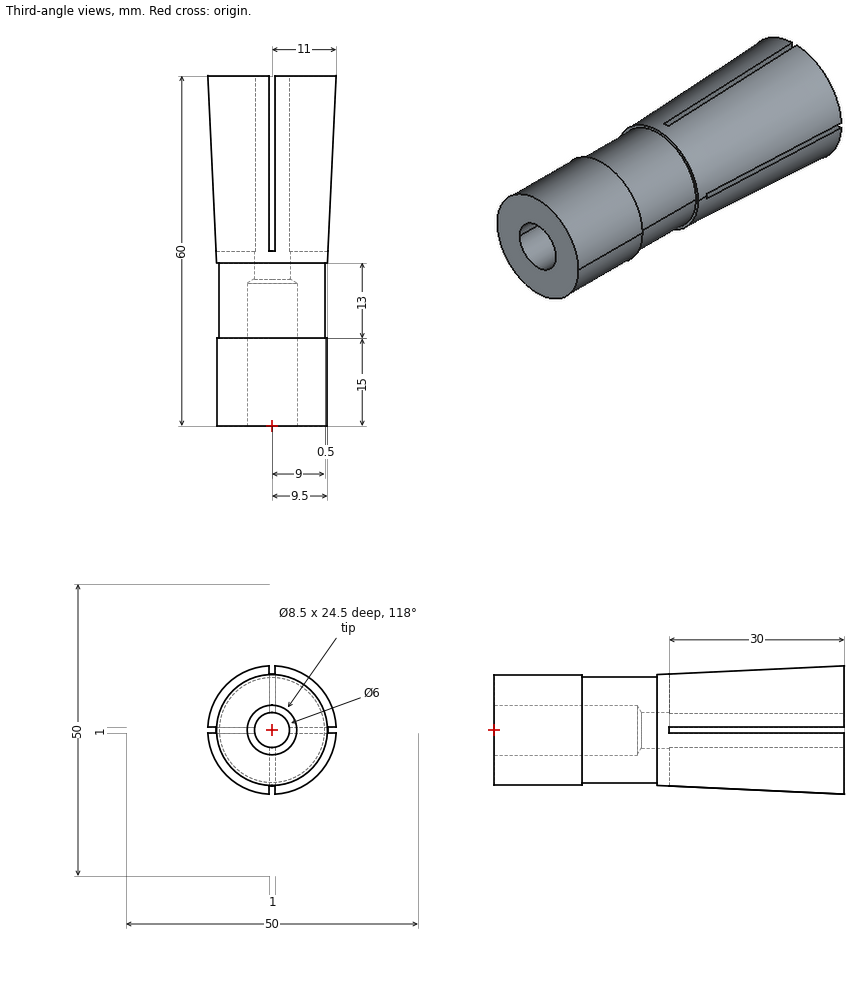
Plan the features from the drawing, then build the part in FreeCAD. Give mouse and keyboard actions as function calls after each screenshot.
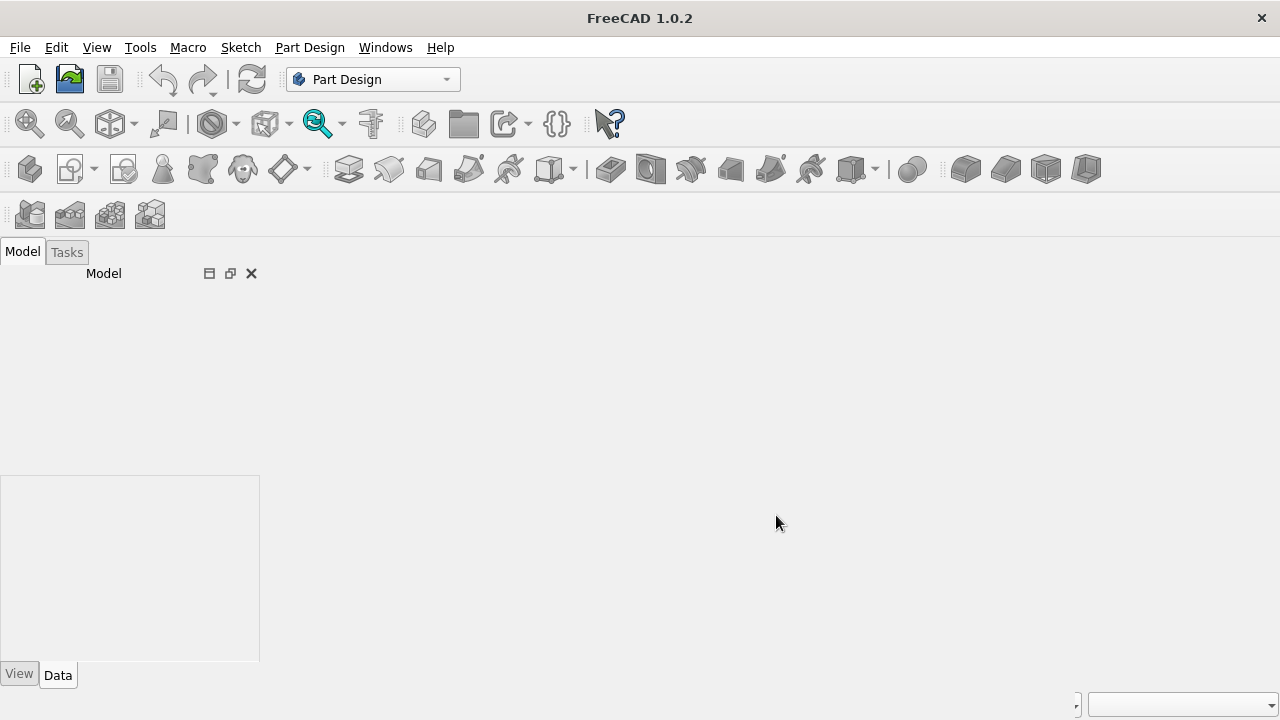
click(30, 80)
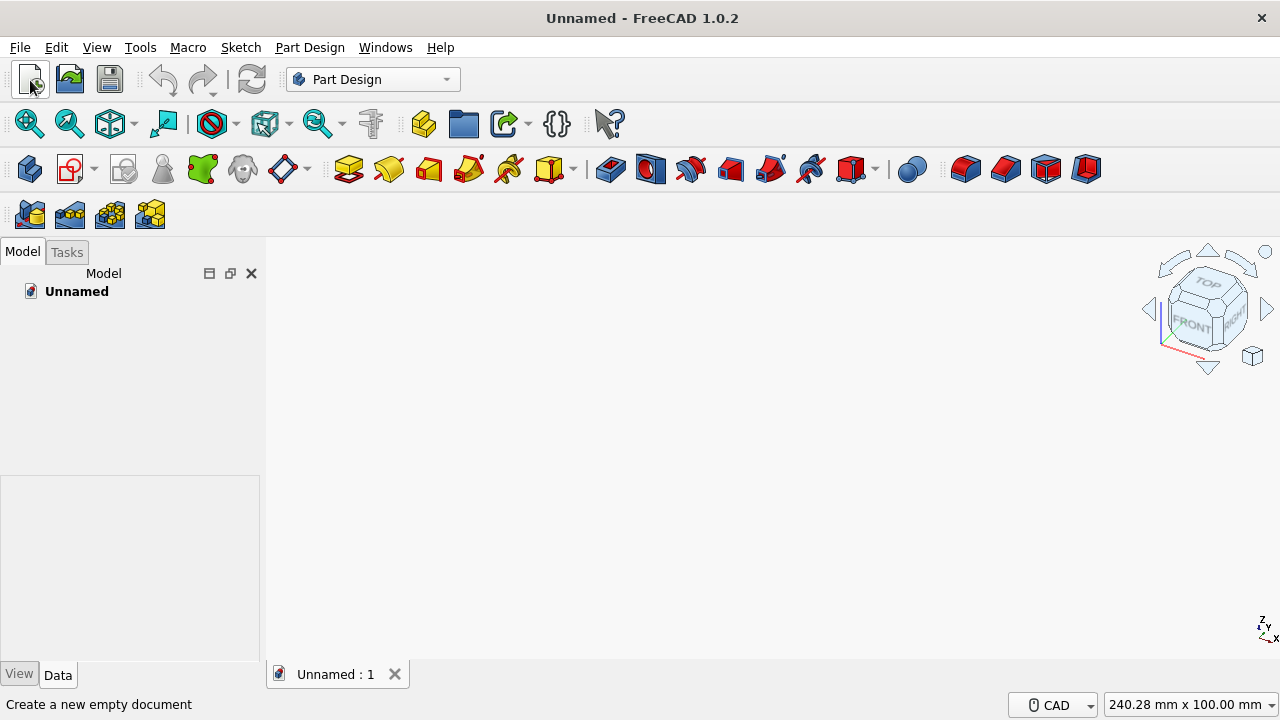
click(70, 170)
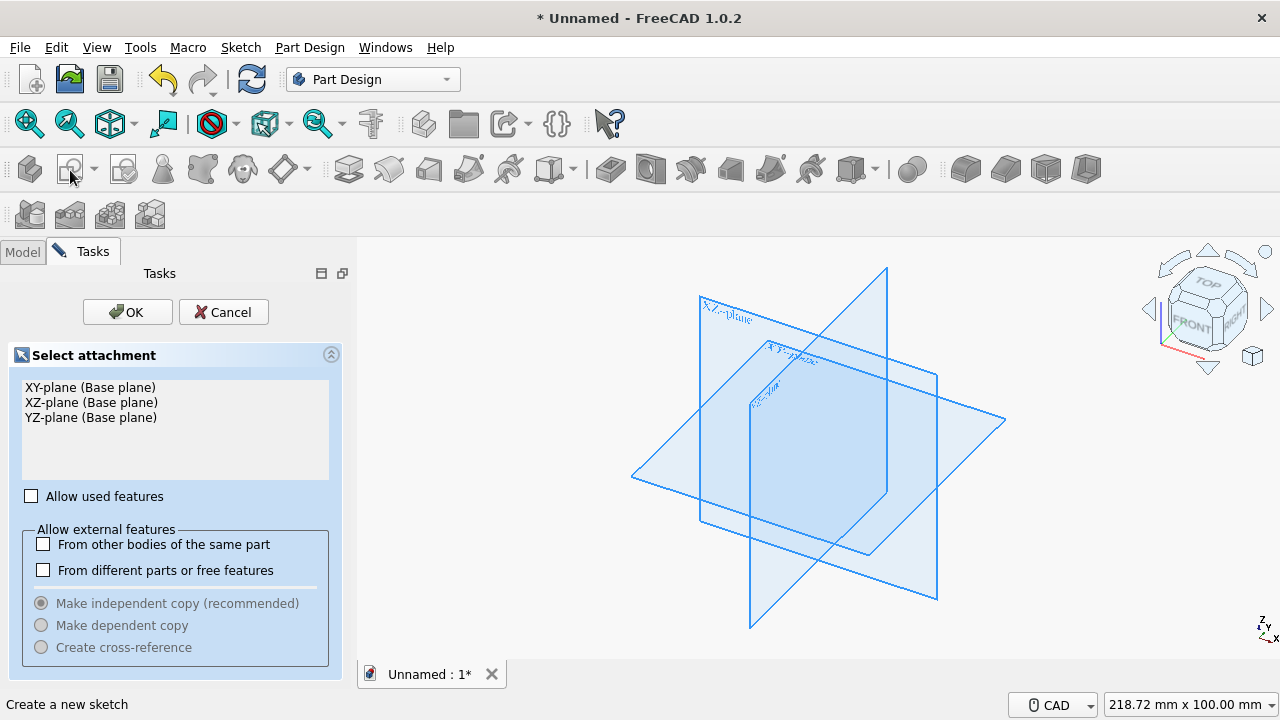
click(82, 388)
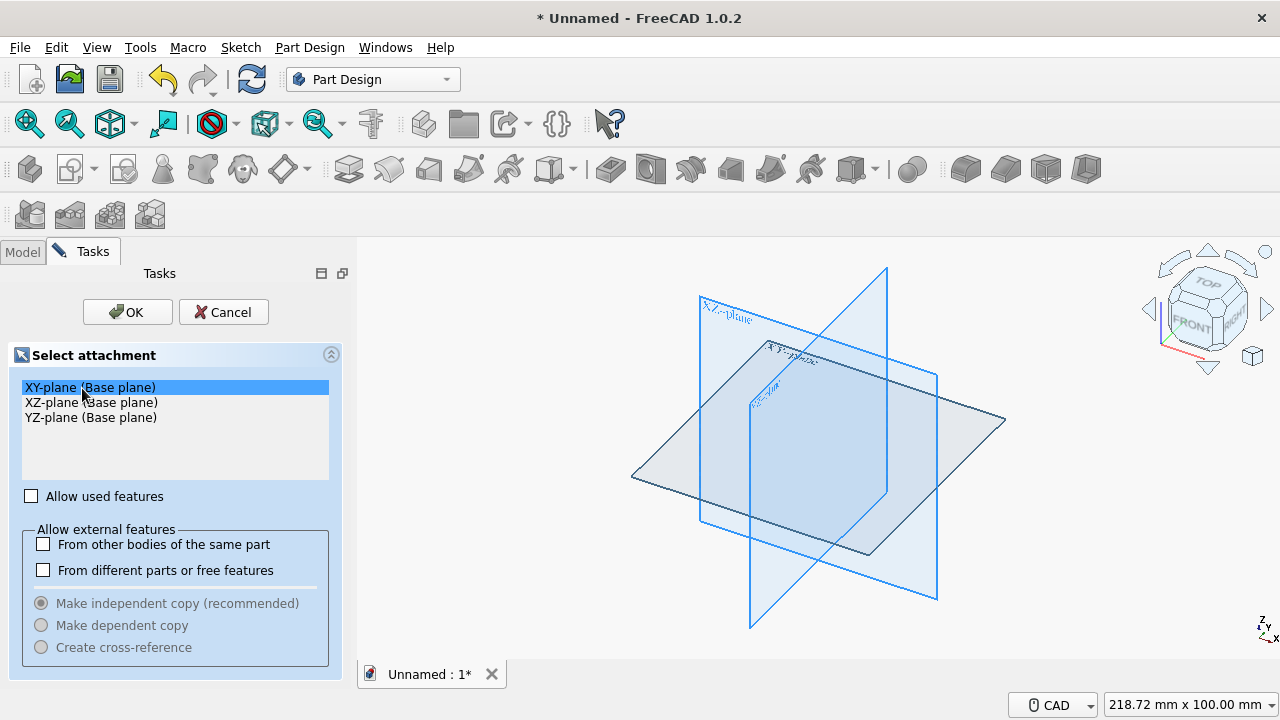
click(128, 312)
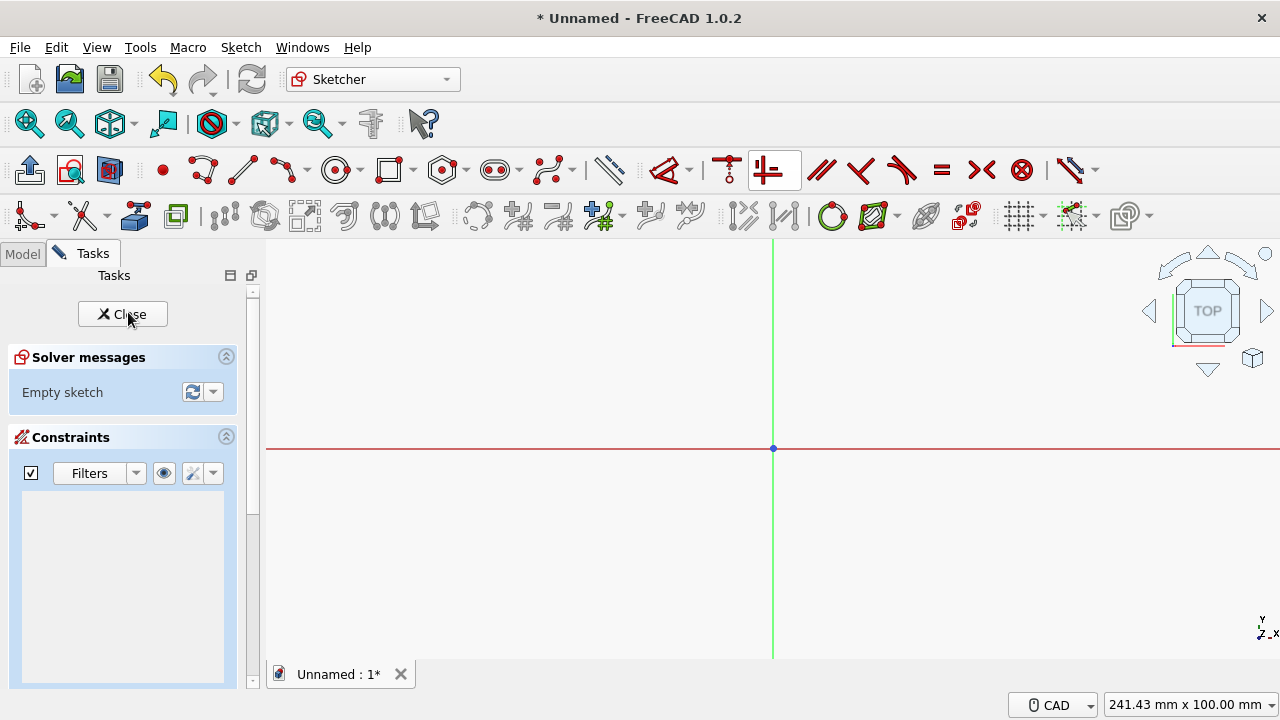
scroll(518, 631, down, 2)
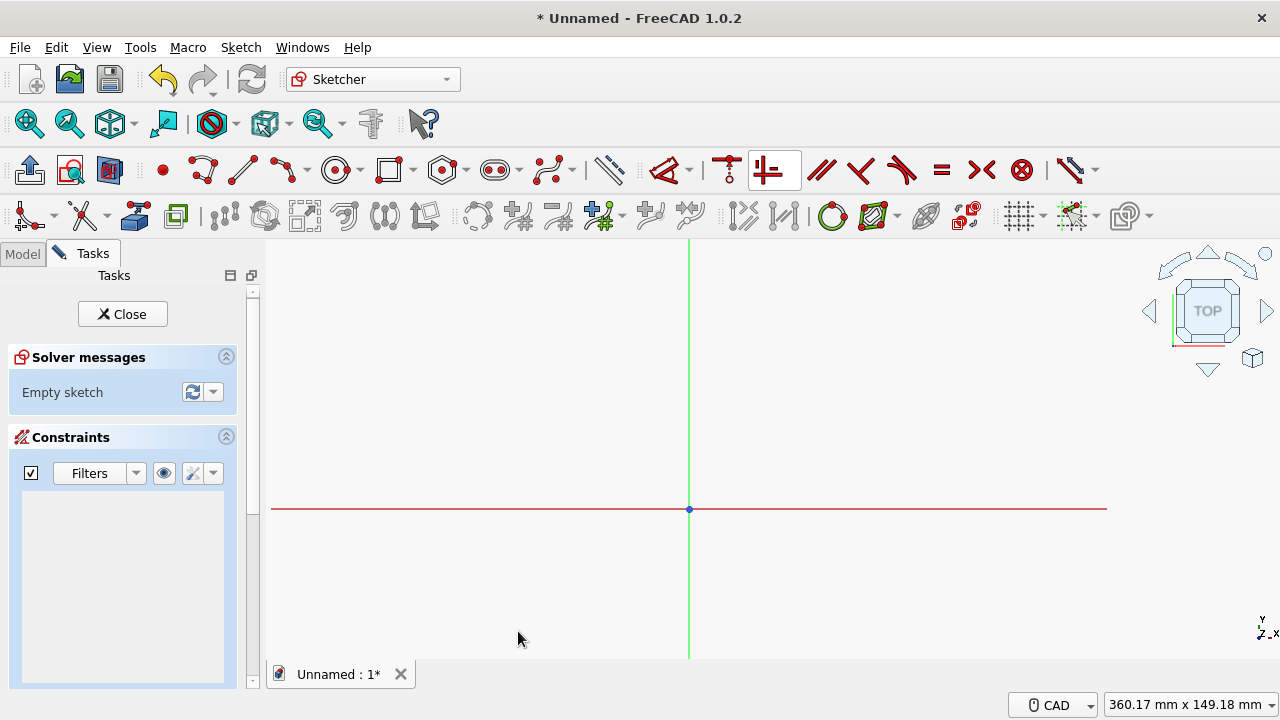
scroll(704, 376, up, 2)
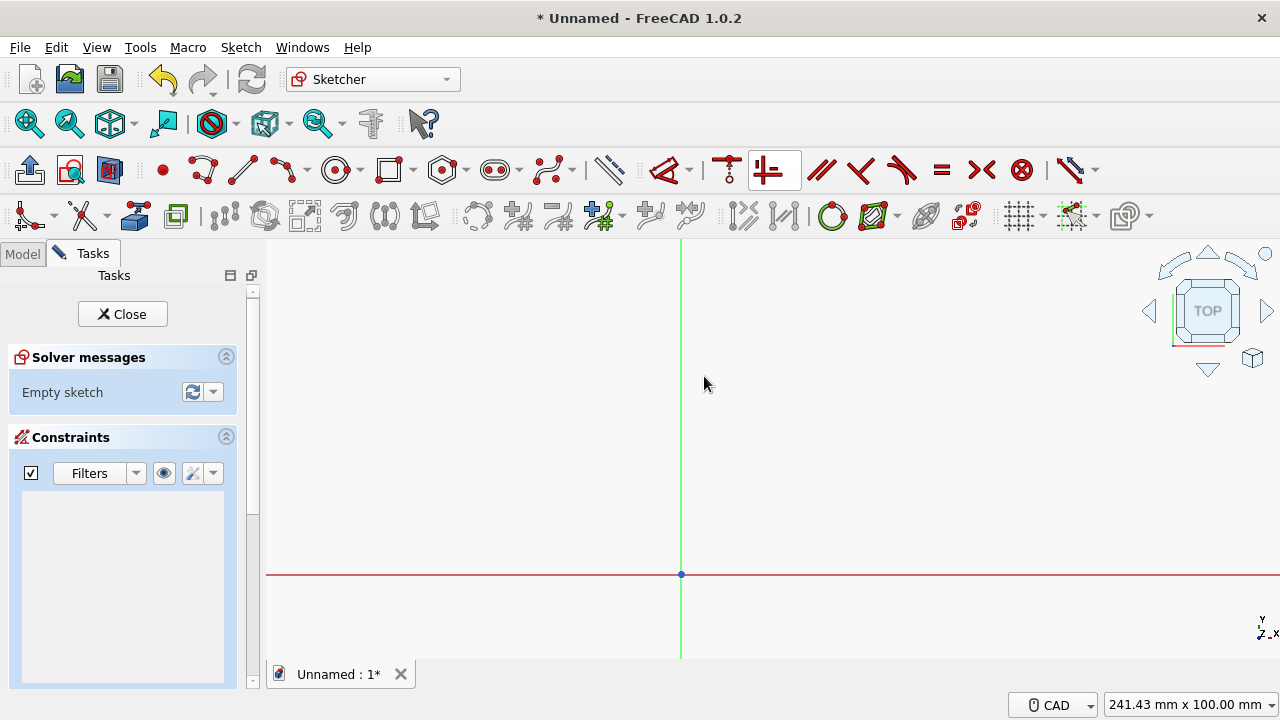
key(g)
key(m)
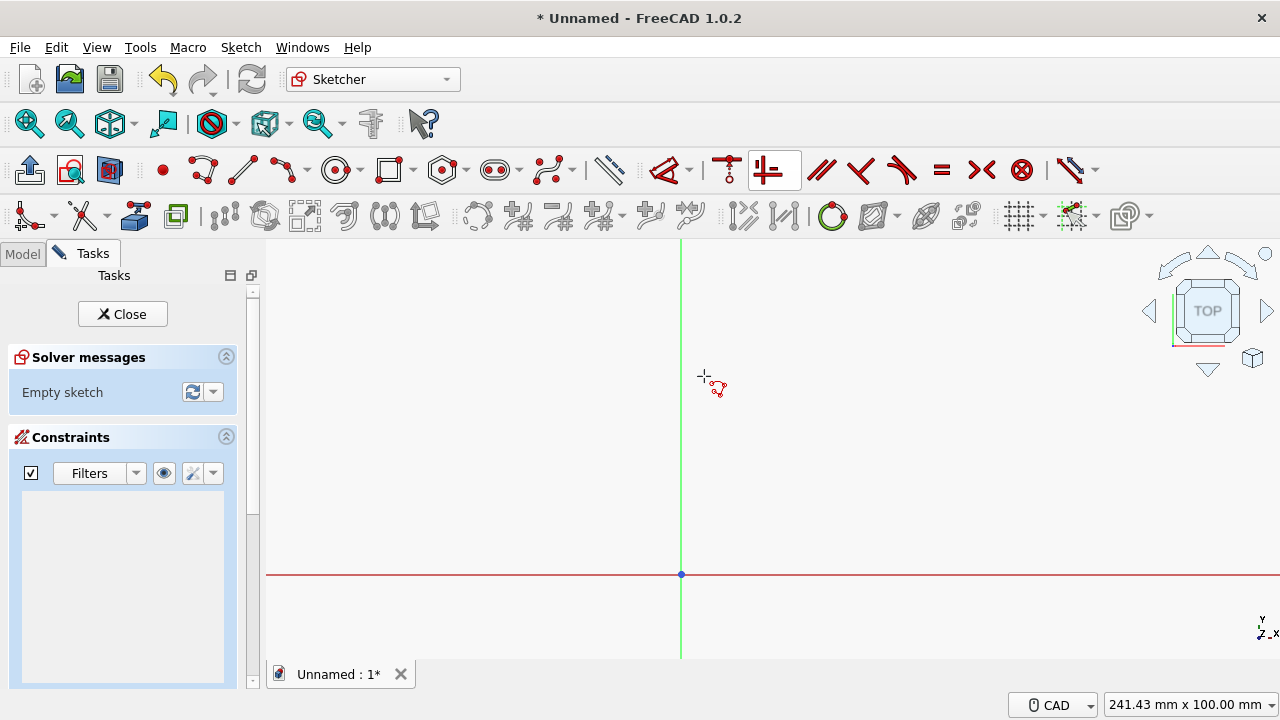
click(681, 575)
click(721, 566)
click(721, 512)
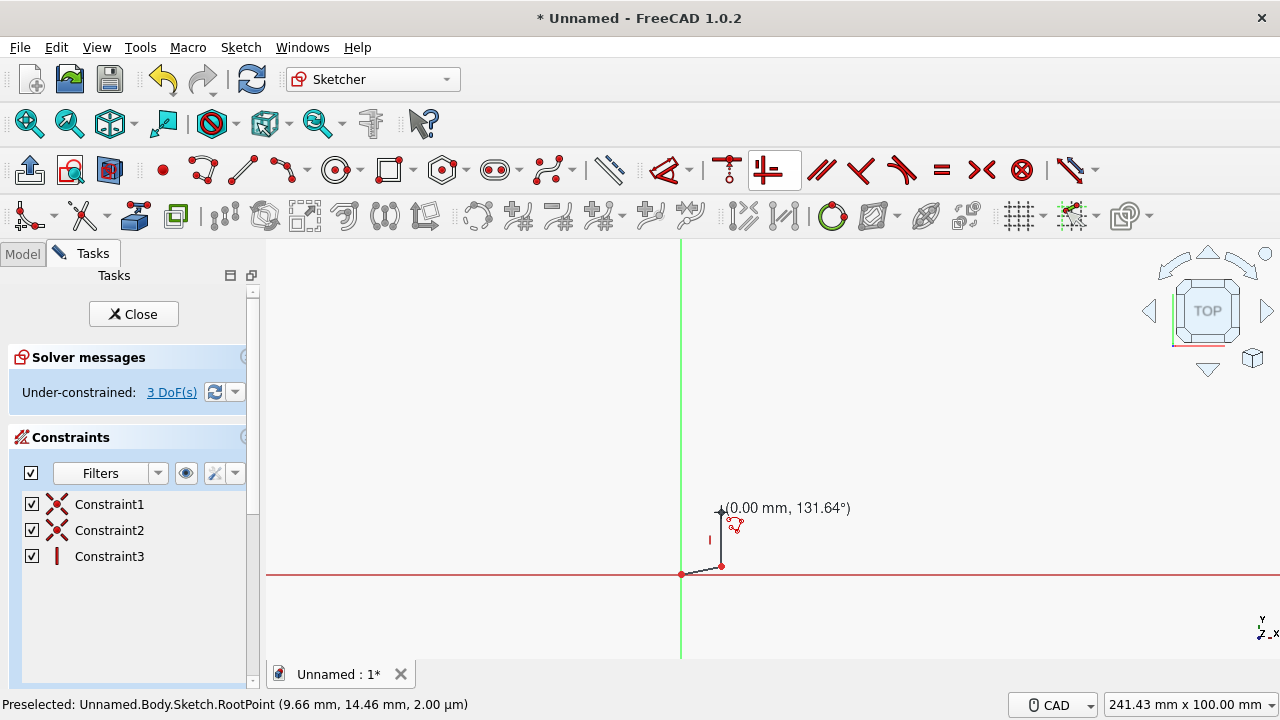
scroll(719, 512, up, 11)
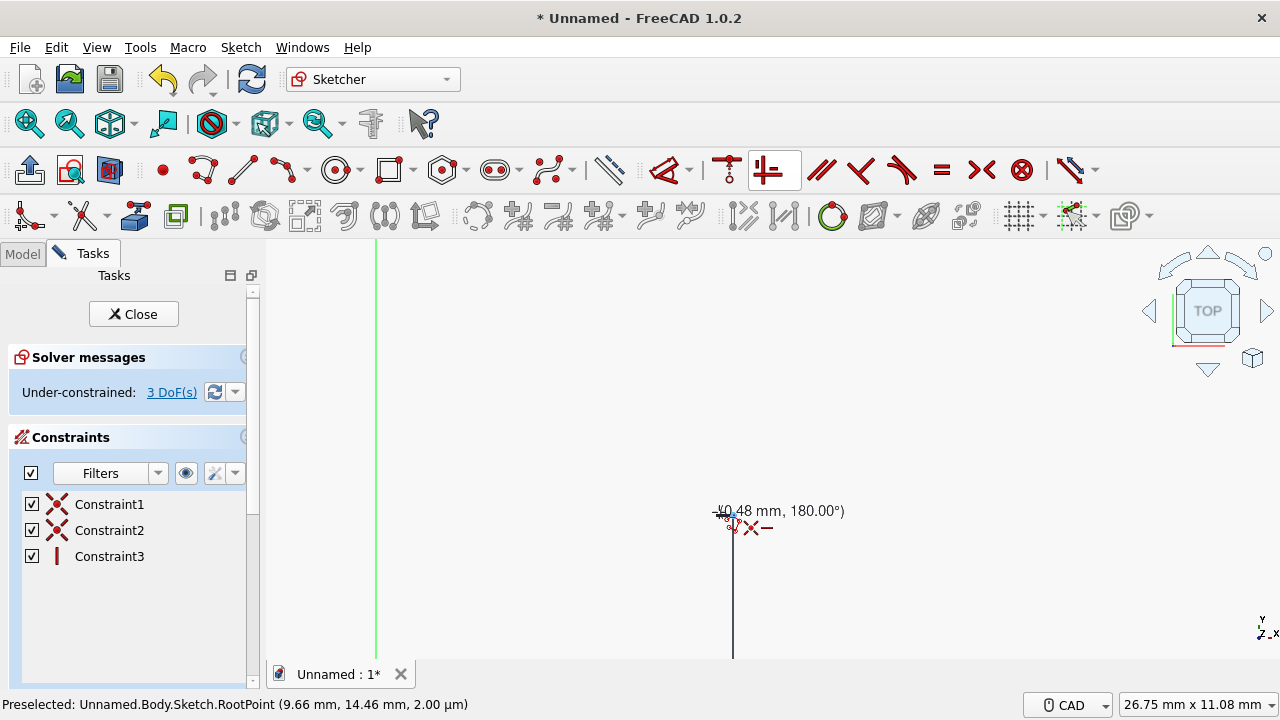
click(717, 507)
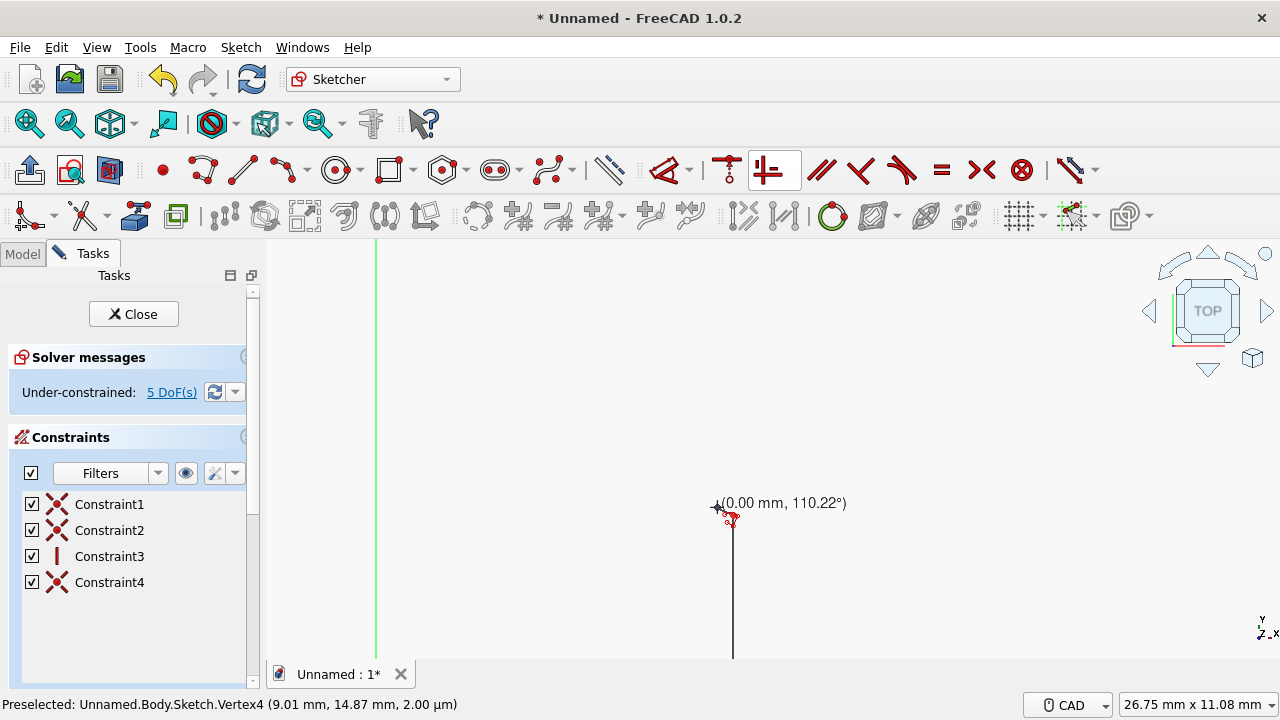
scroll(719, 513, down, 11)